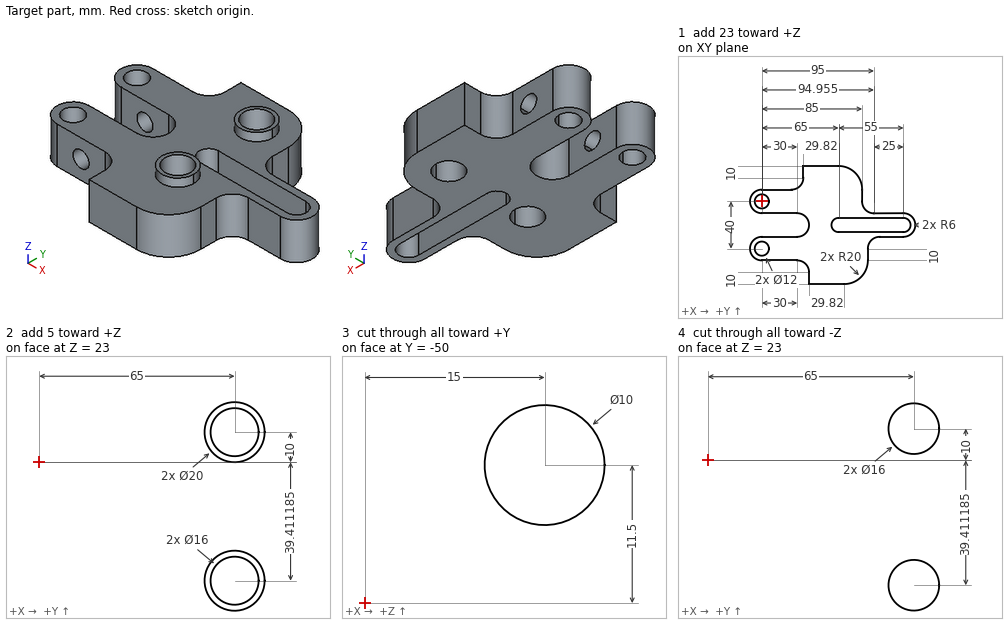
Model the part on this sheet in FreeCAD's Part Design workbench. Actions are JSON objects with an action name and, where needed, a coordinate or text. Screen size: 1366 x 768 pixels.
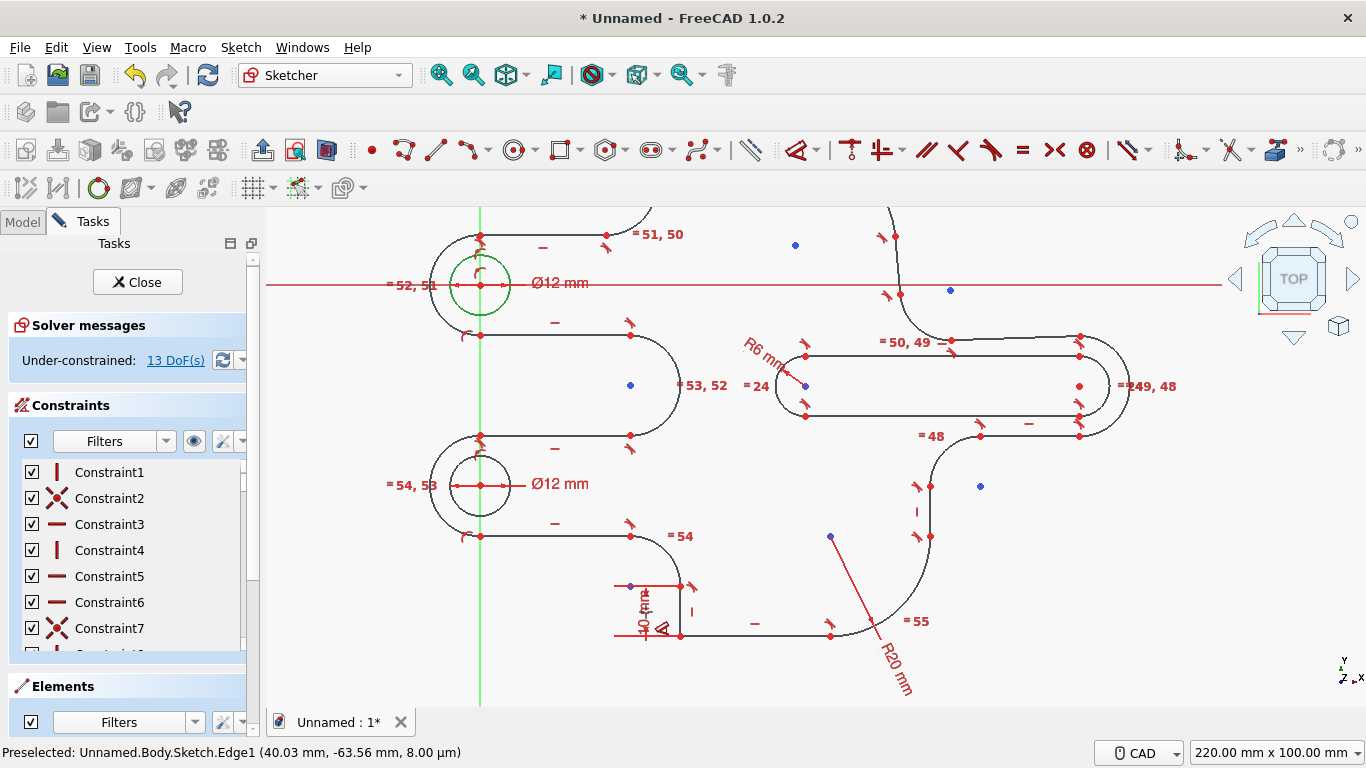
{"action": "left_click", "coordinate": [930, 521]}
{"action": "left_click", "coordinate": [964, 511]}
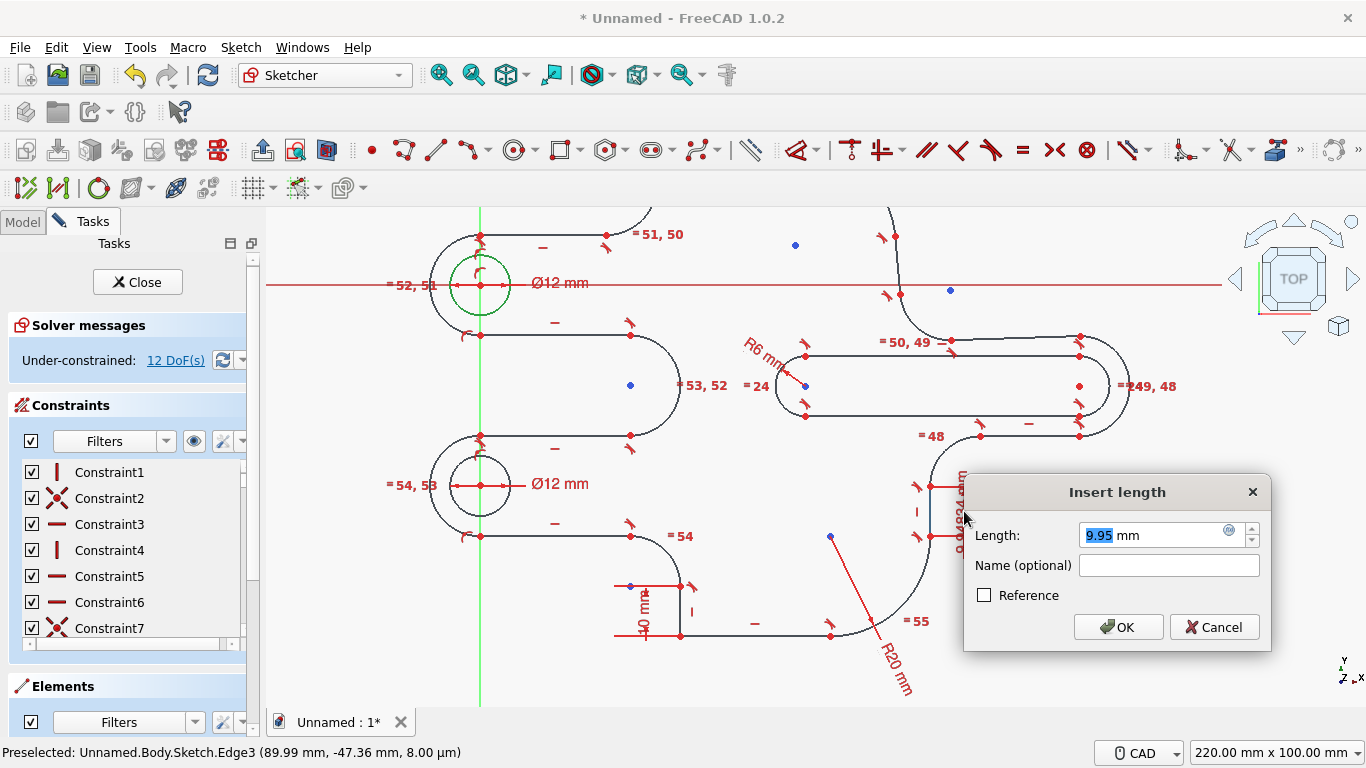
{"action": "type", "text": "10"}
{"action": "key", "text": "Return"}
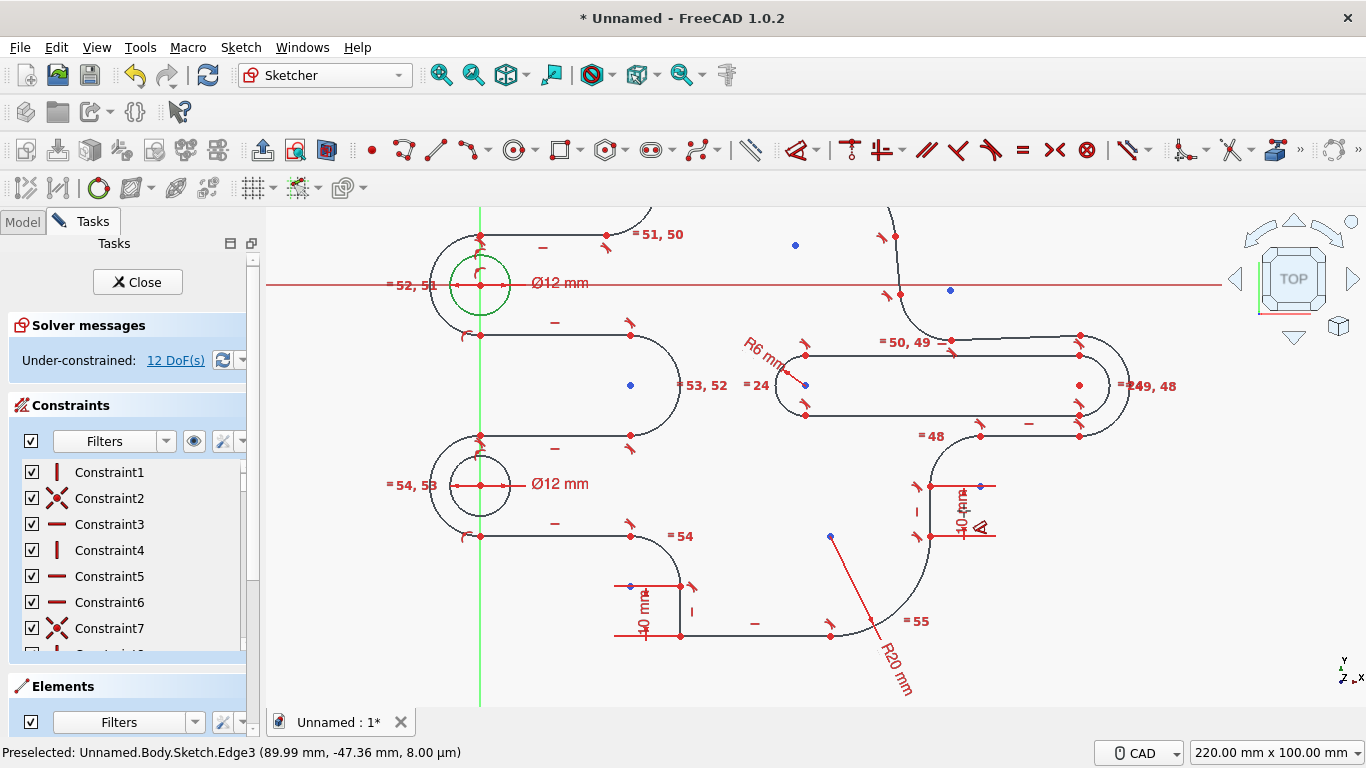
{"action": "scroll", "coordinate": [681, 603], "scroll_direction": "down", "scroll_amount": 2}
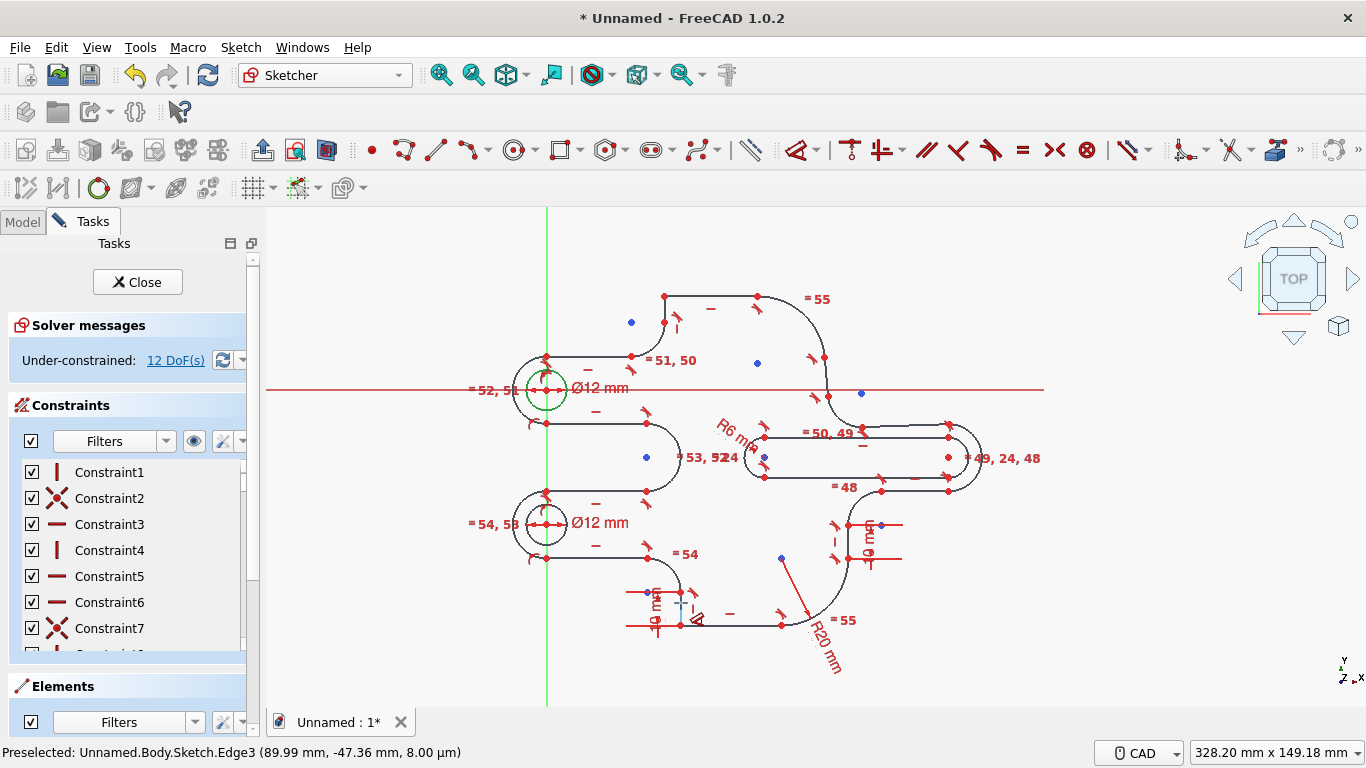
{"action": "scroll", "coordinate": [665, 304], "scroll_direction": "up", "scroll_amount": 3}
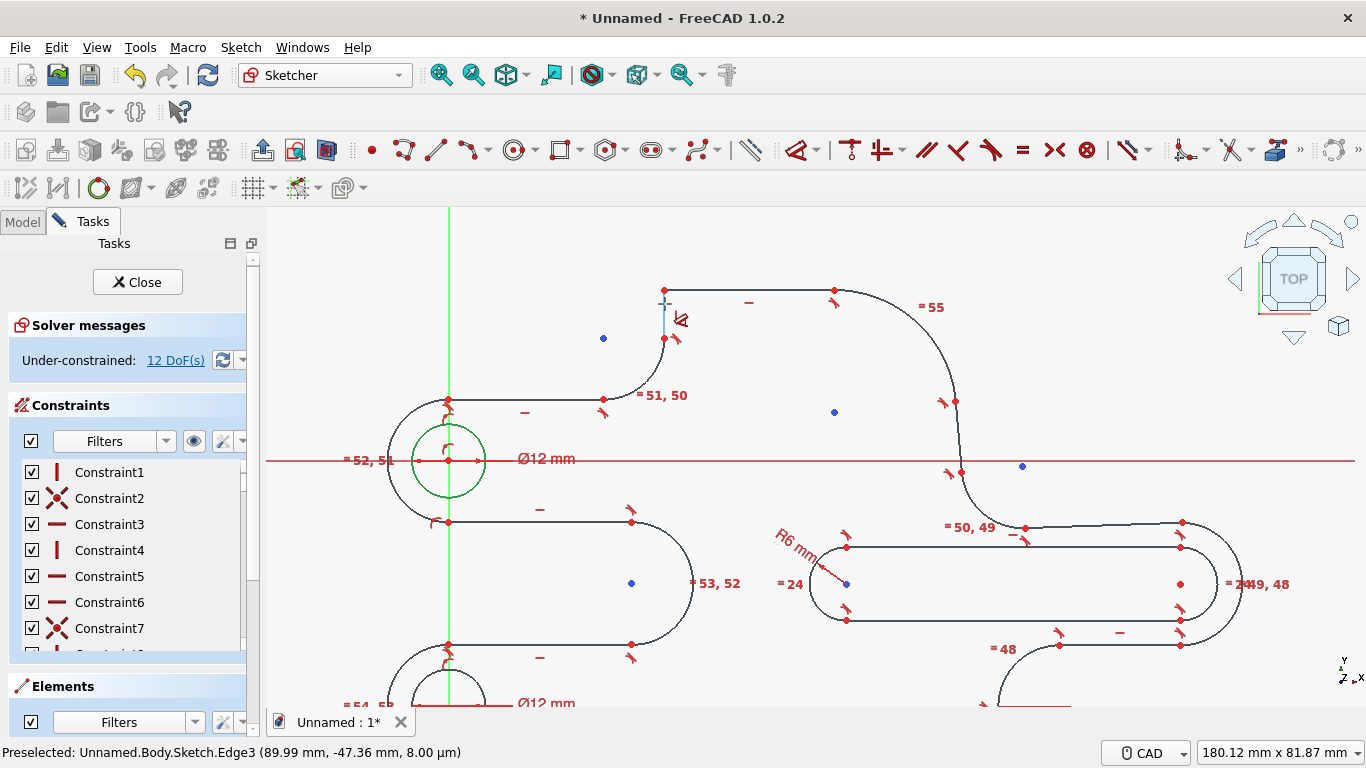
{"action": "left_click", "coordinate": [664, 305]}
{"action": "left_click", "coordinate": [630, 314]}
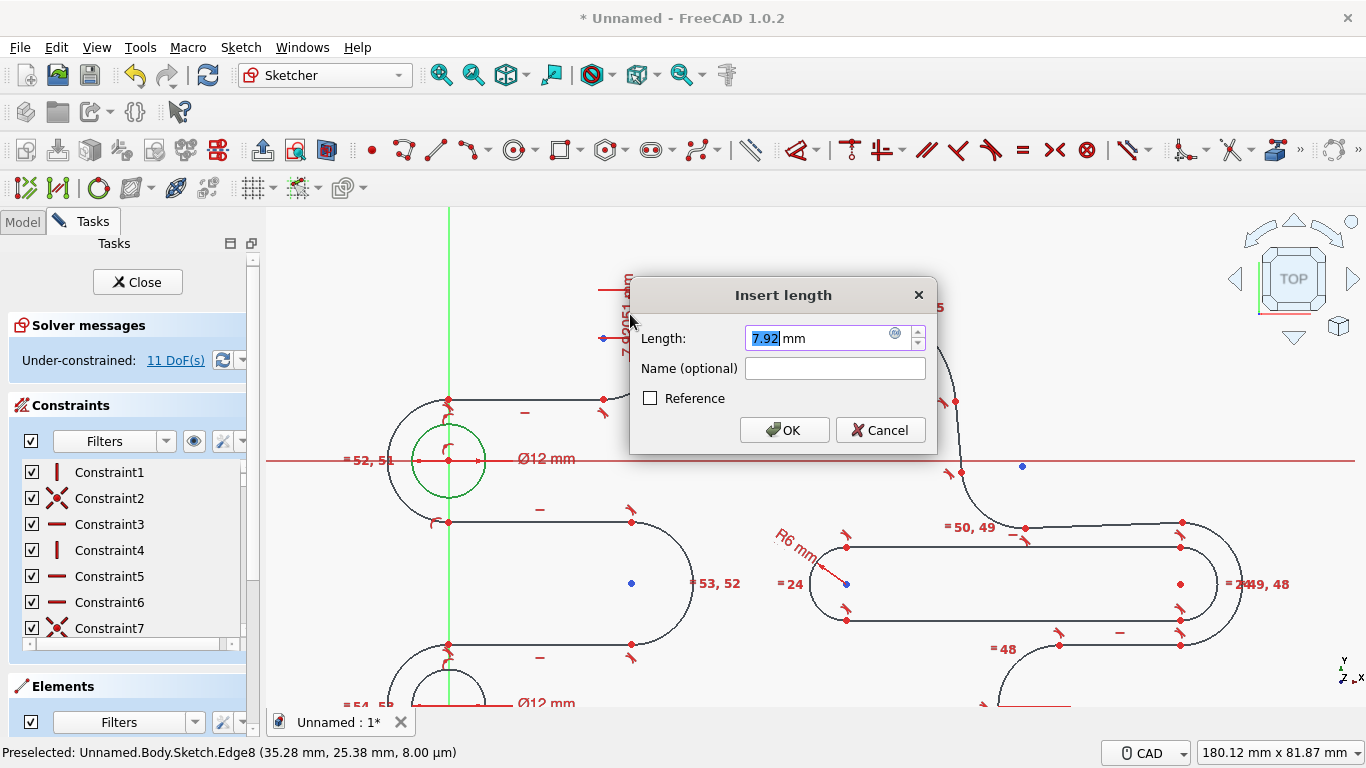
{"action": "type", "text": "10"}
{"action": "key", "text": "Return"}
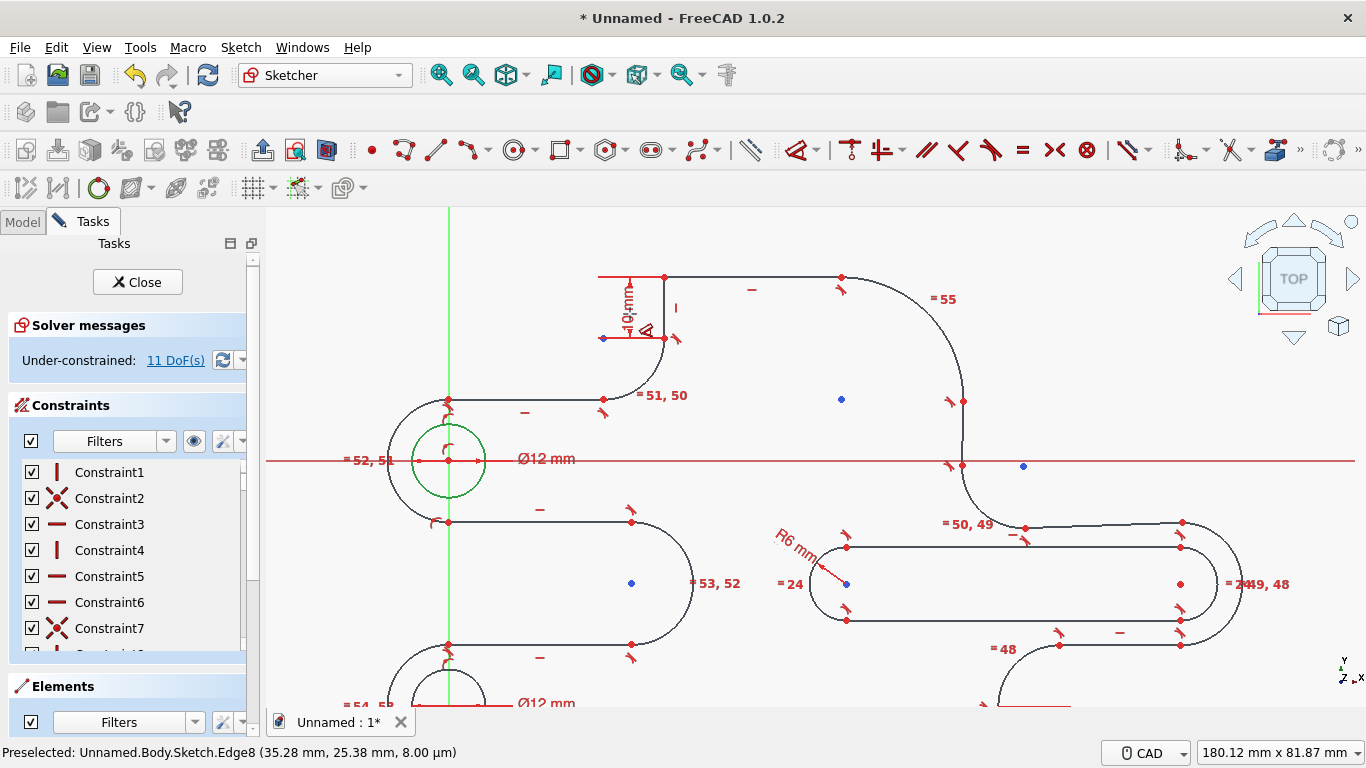
{"action": "left_click", "coordinate": [504, 522]}
{"action": "left_click", "coordinate": [540, 488]}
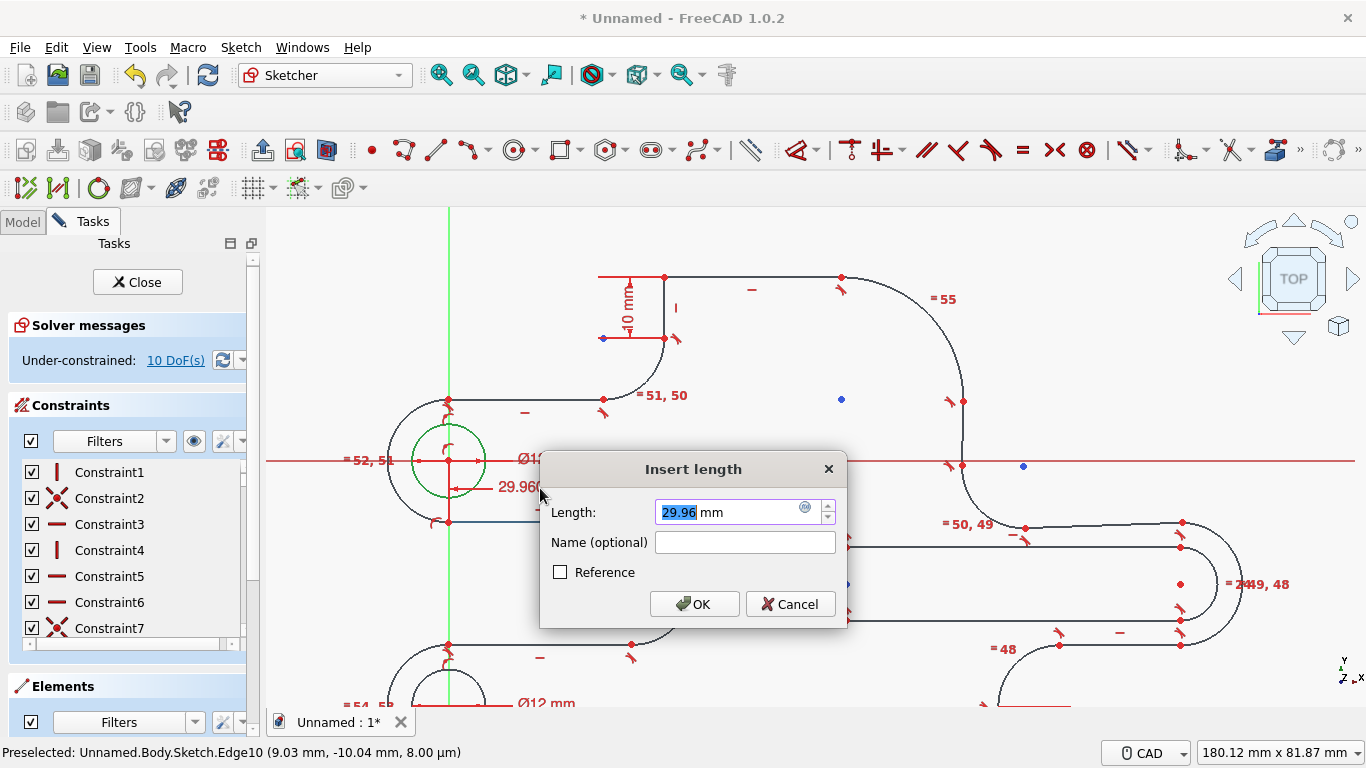
{"action": "type", "text": "30"}
{"action": "key", "text": "Return"}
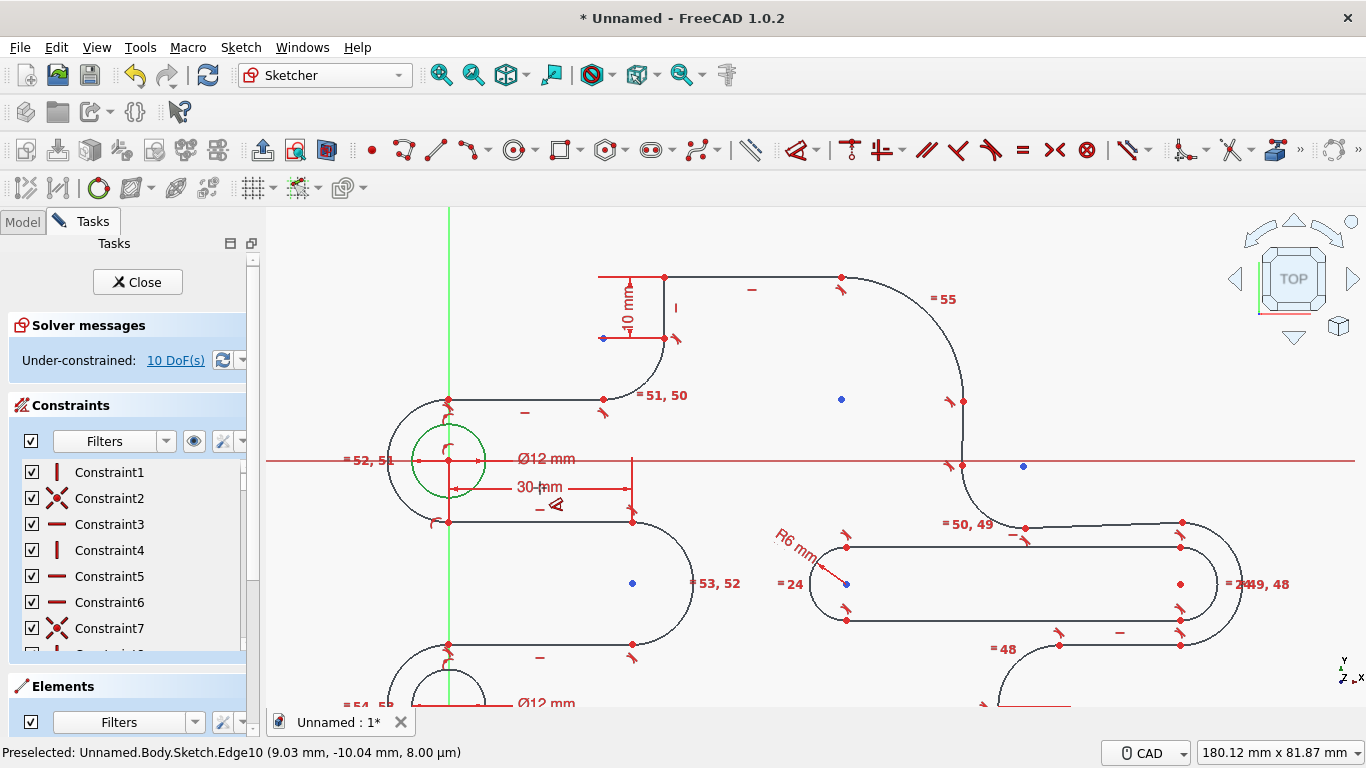
{"action": "scroll", "coordinate": [665, 304], "scroll_direction": "down", "scroll_amount": 3}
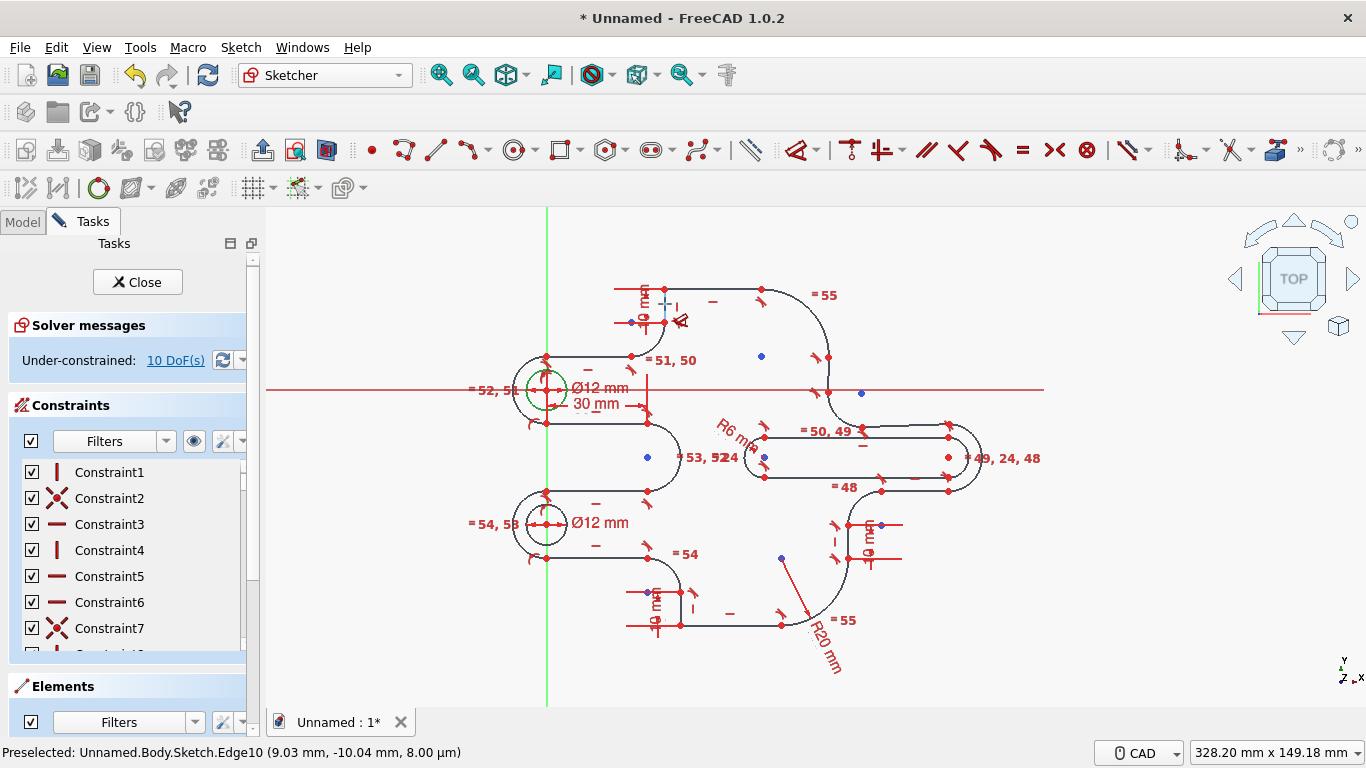
{"action": "left_click", "coordinate": [577, 558]}
{"action": "left_click", "coordinate": [574, 592]}